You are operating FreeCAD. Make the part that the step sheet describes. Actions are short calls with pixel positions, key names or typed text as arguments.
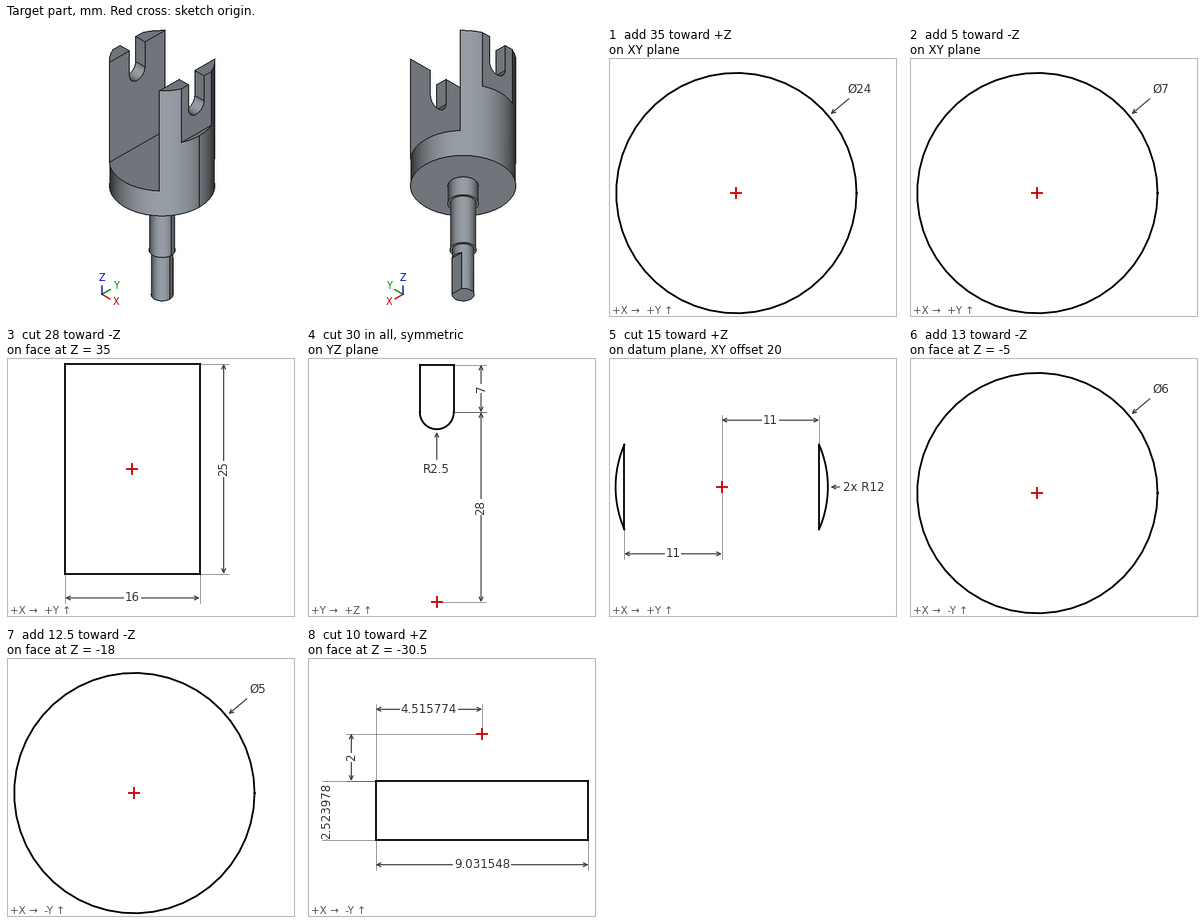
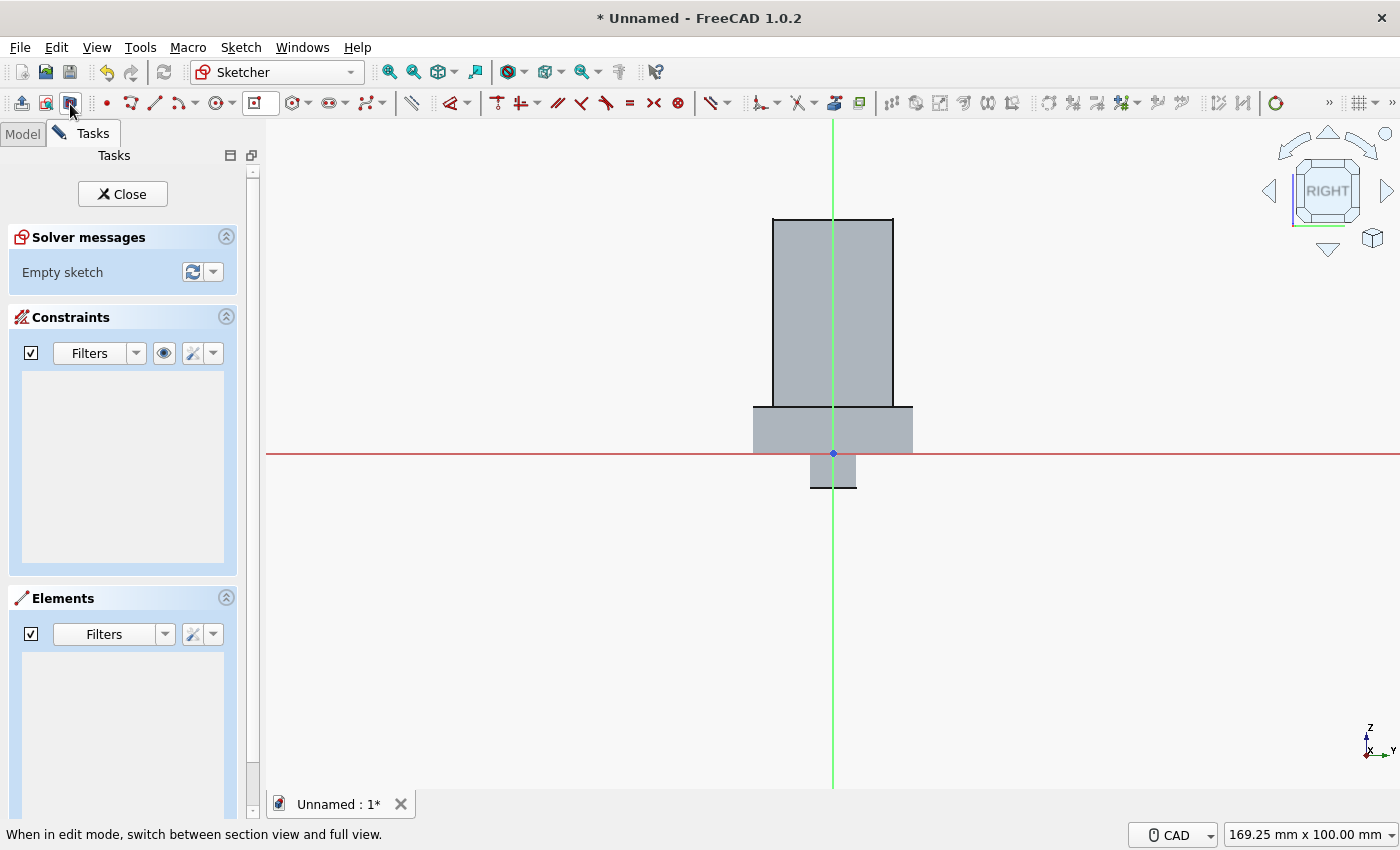
scroll(844, 220, up, 10)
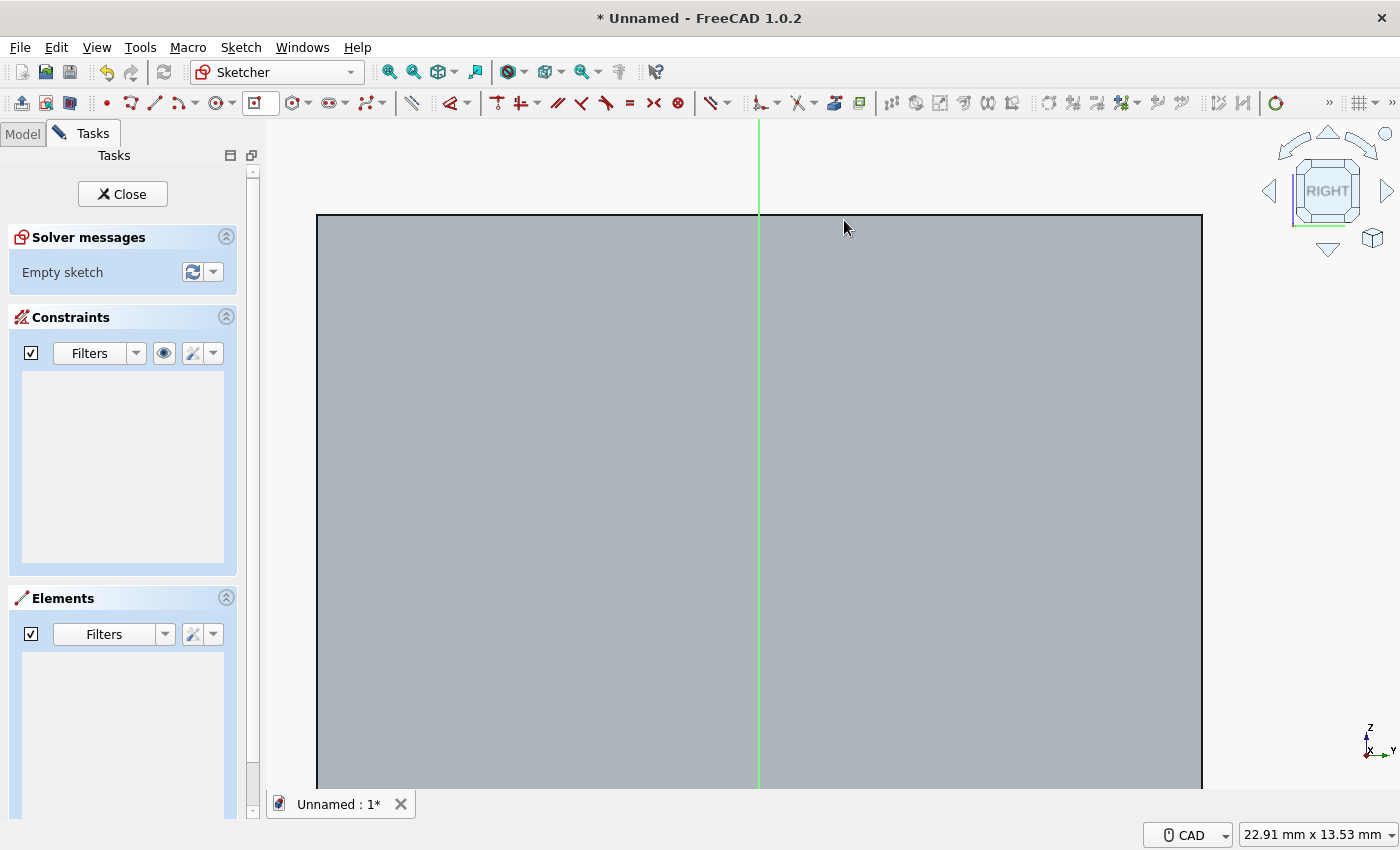
click(132, 104)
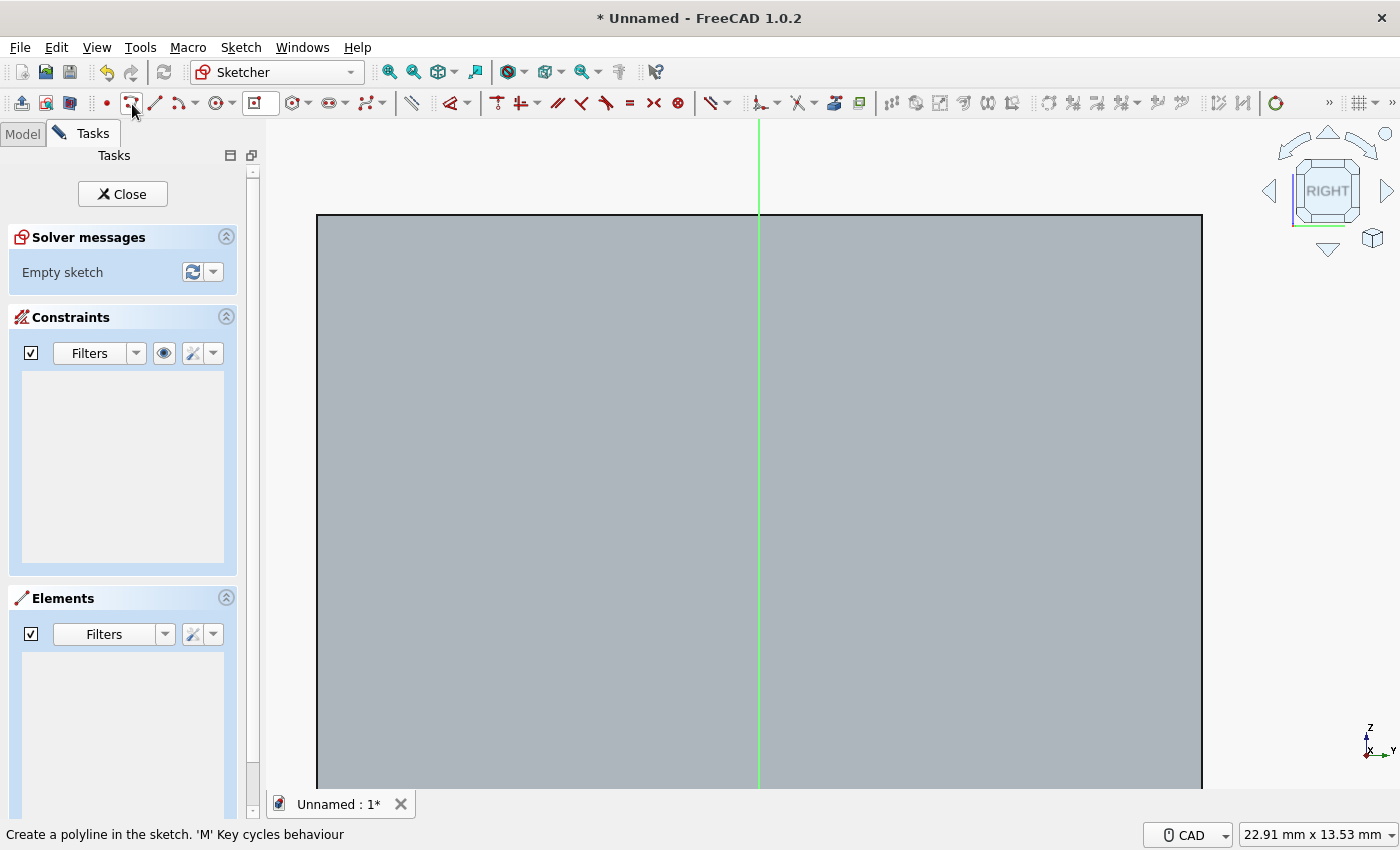
click(883, 562)
click(883, 215)
click(636, 215)
click(636, 562)
right_click(636, 562)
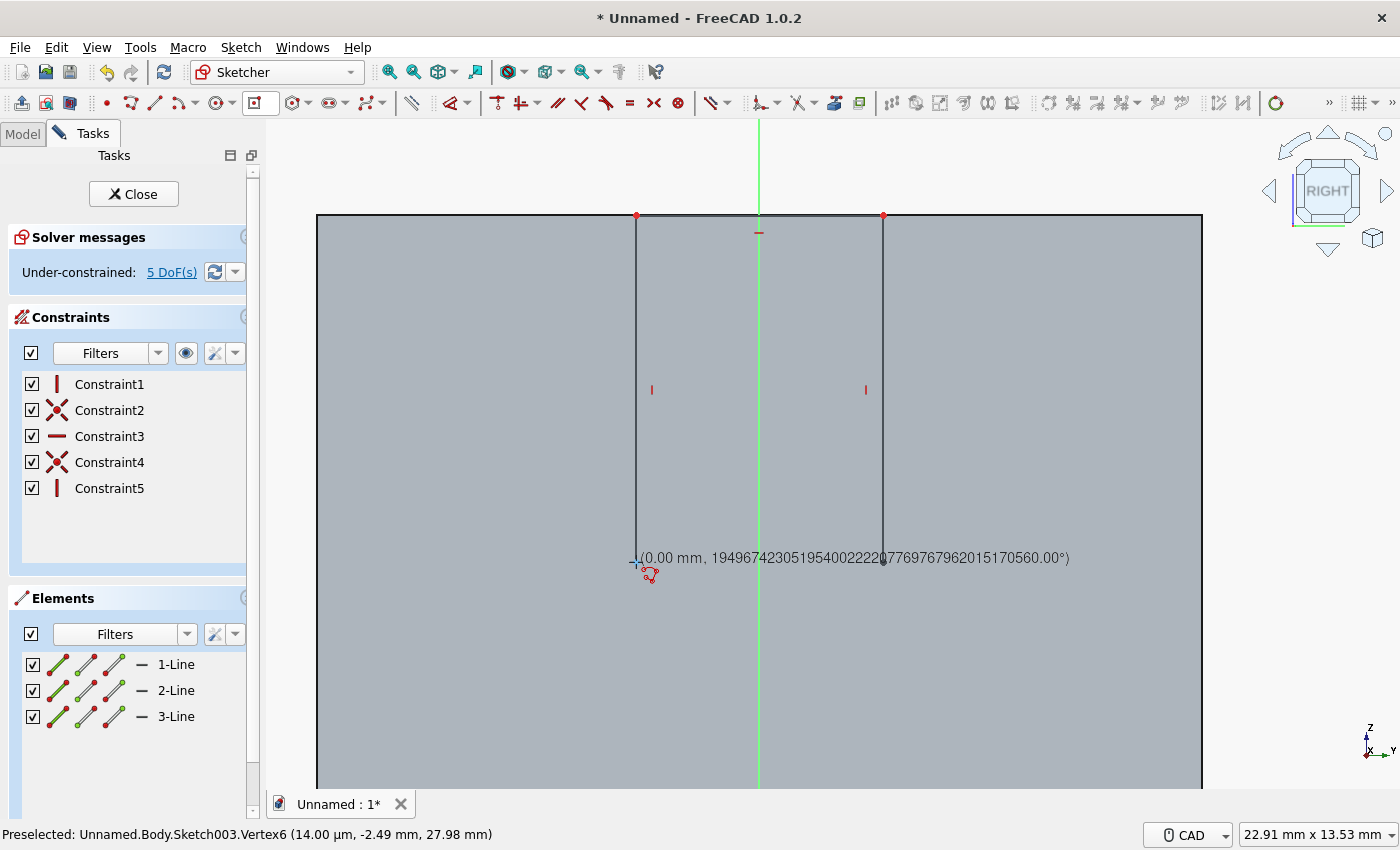
key(g)
key(3)
key(a)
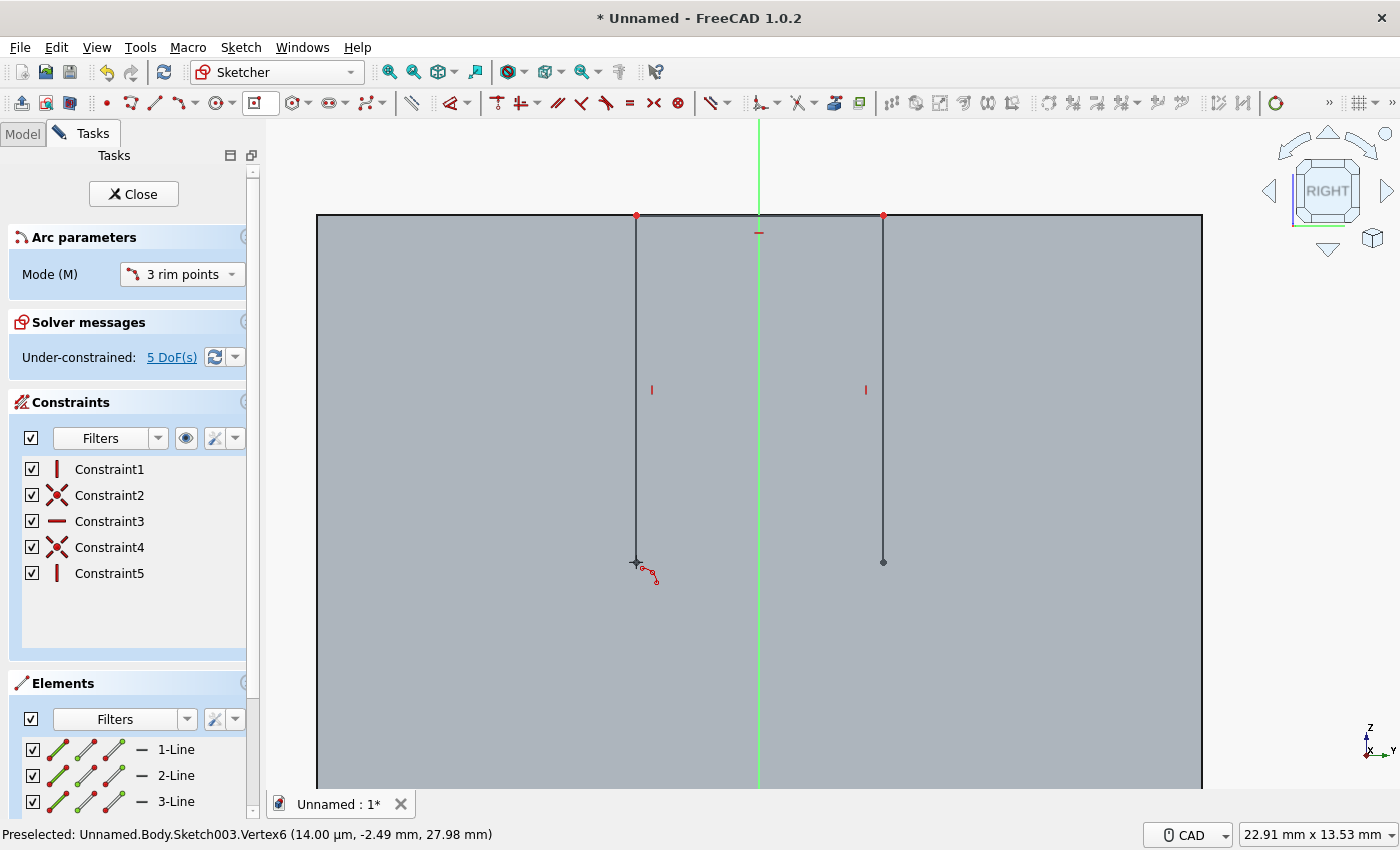
click(636, 563)
click(883, 563)
click(721, 680)
key(Escape)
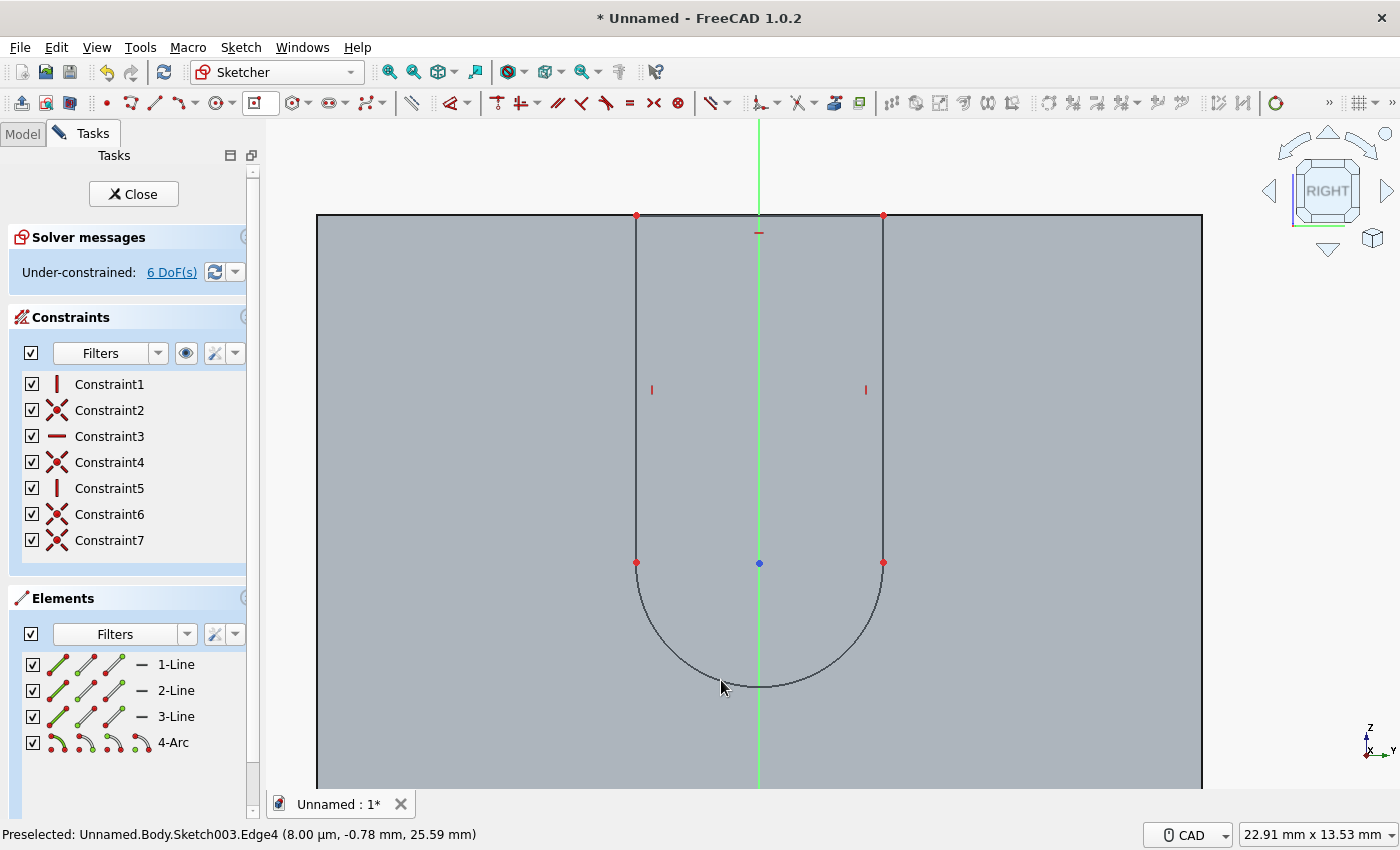
click(883, 459)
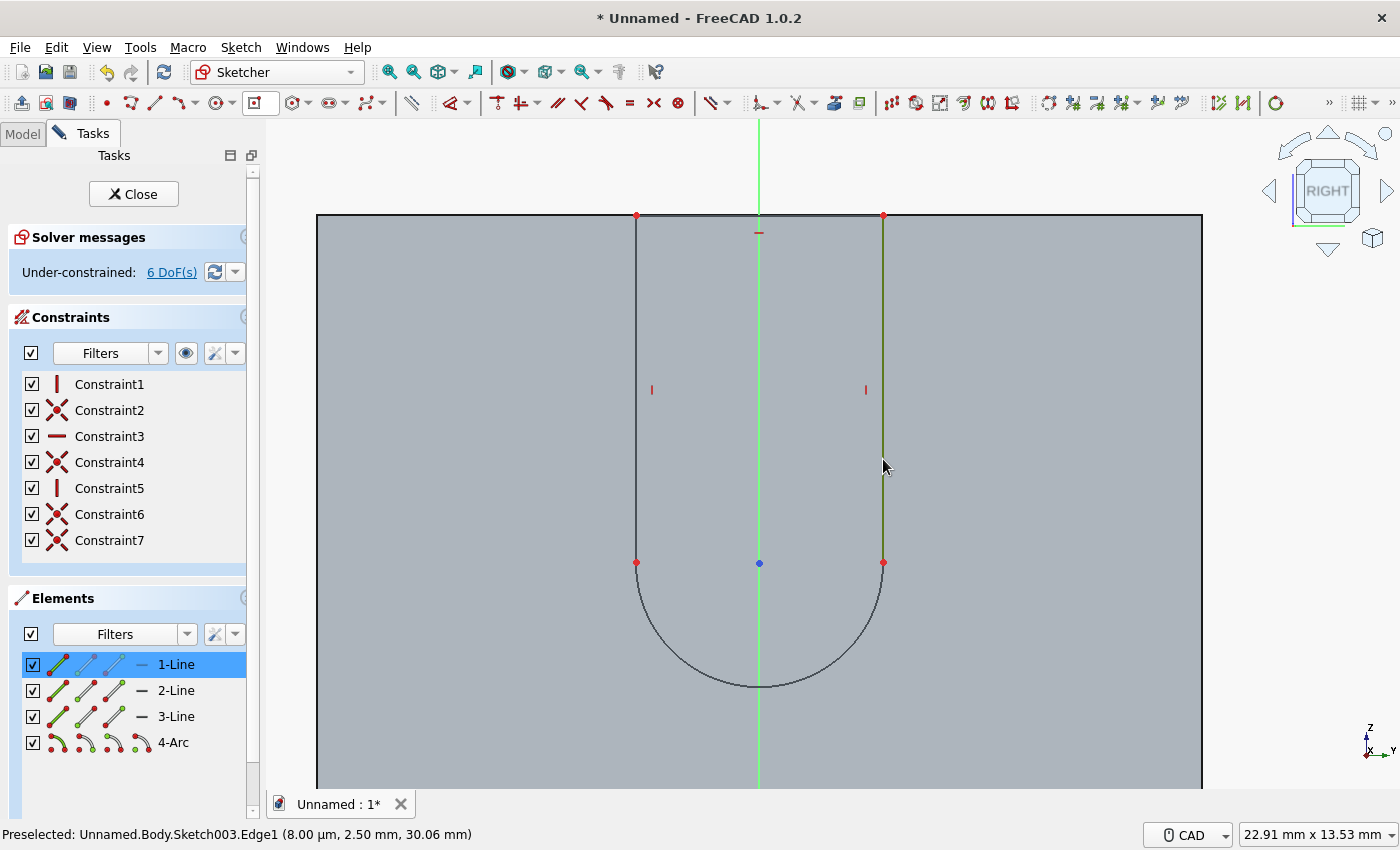
click(687, 663)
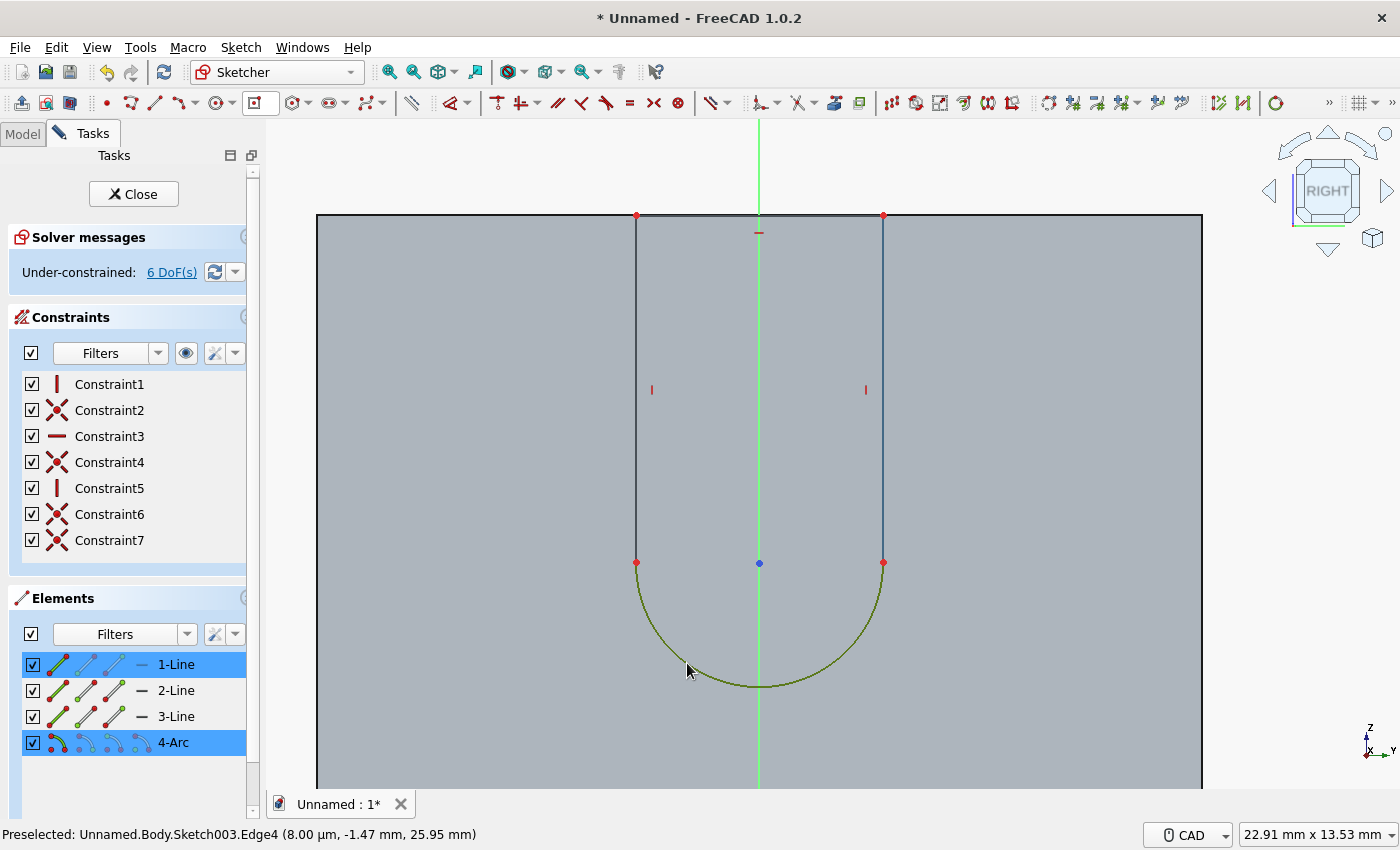
key(t)